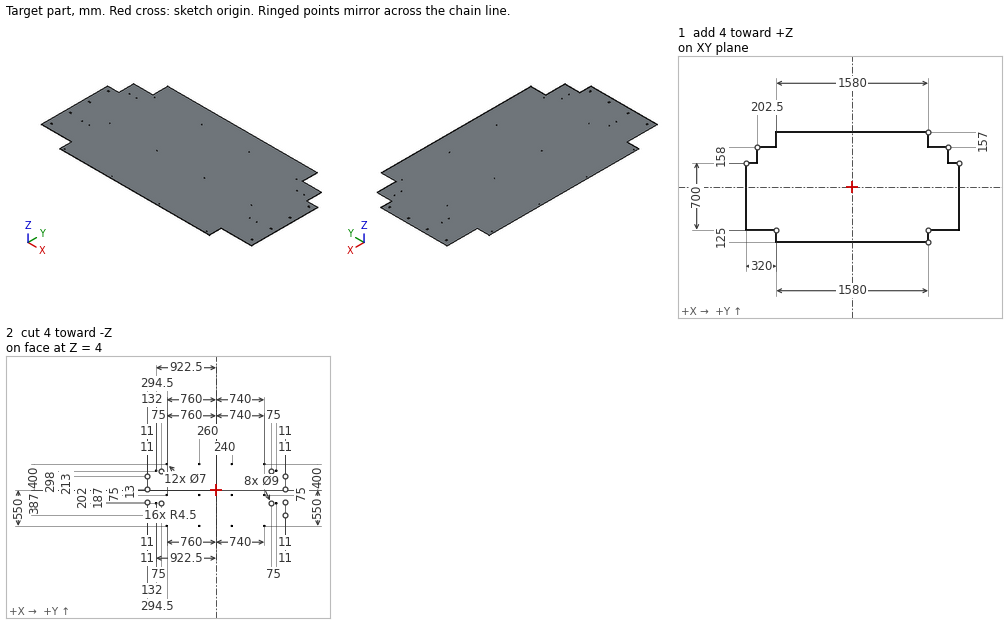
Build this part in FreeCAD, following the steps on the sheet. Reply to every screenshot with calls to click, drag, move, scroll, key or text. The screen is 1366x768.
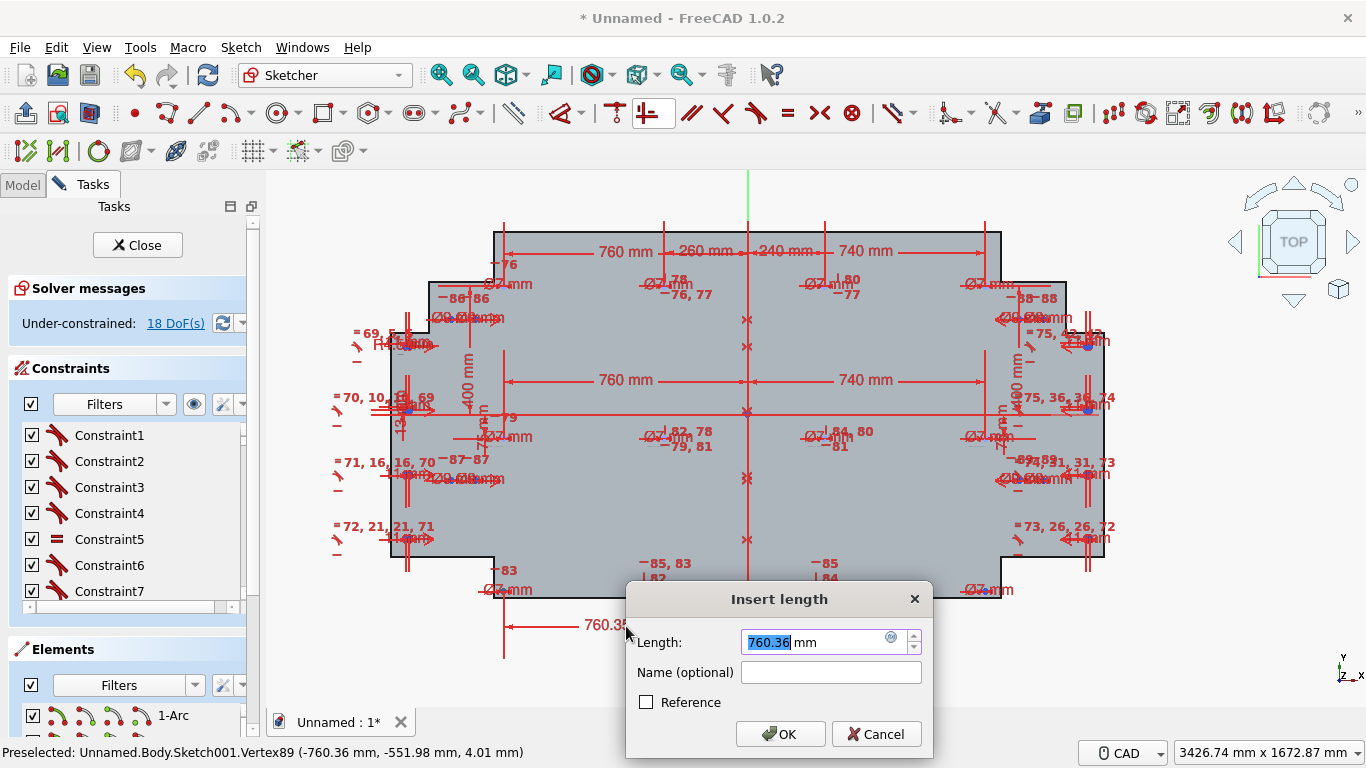
text(760)
key(Return)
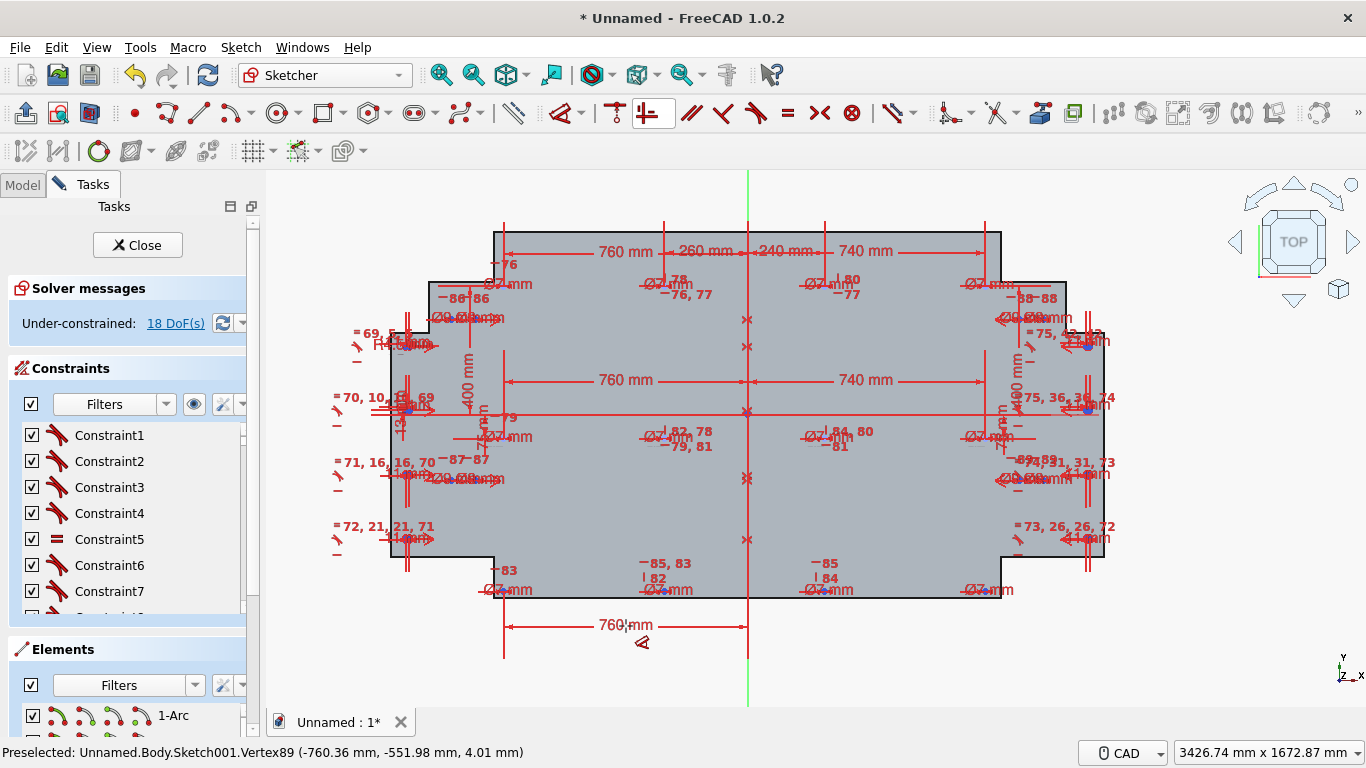
click(504, 592)
click(470, 503)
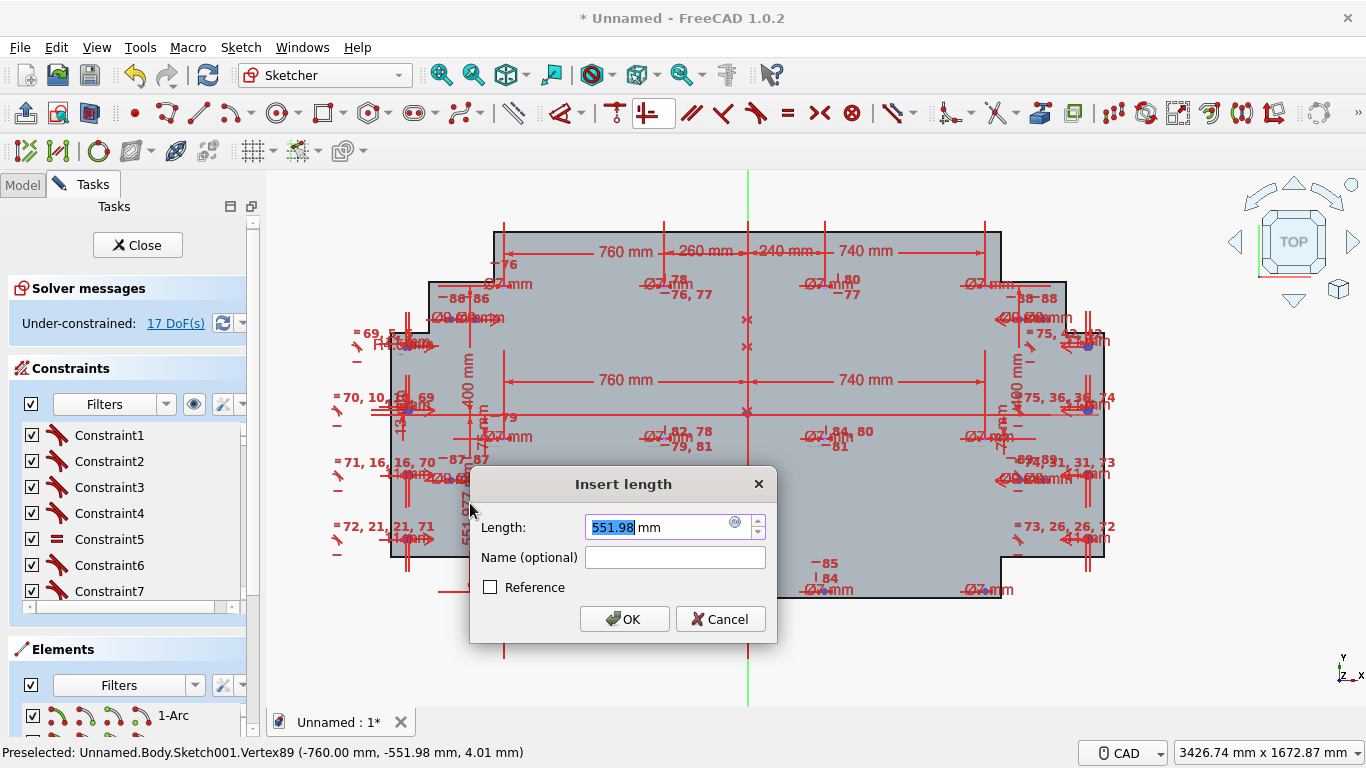
text(550)
key(Return)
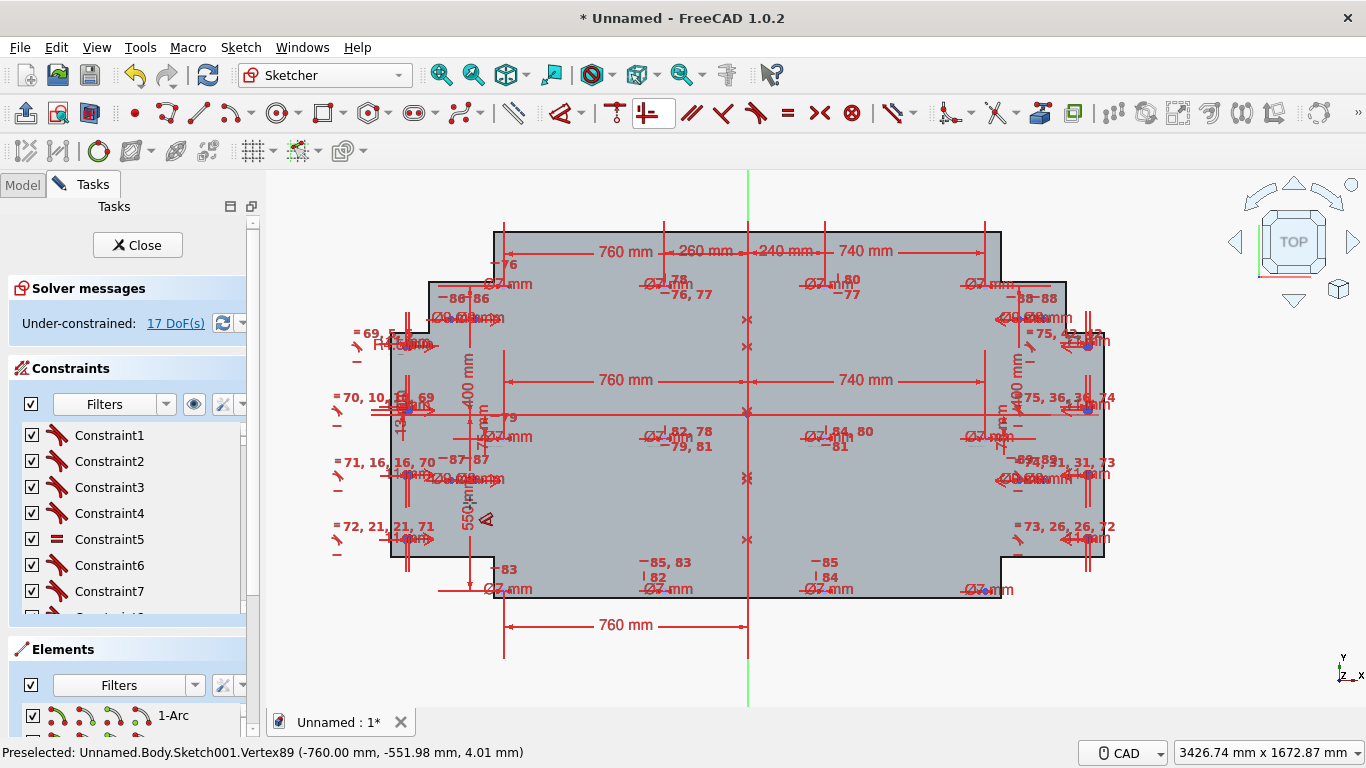
click(985, 592)
click(866, 626)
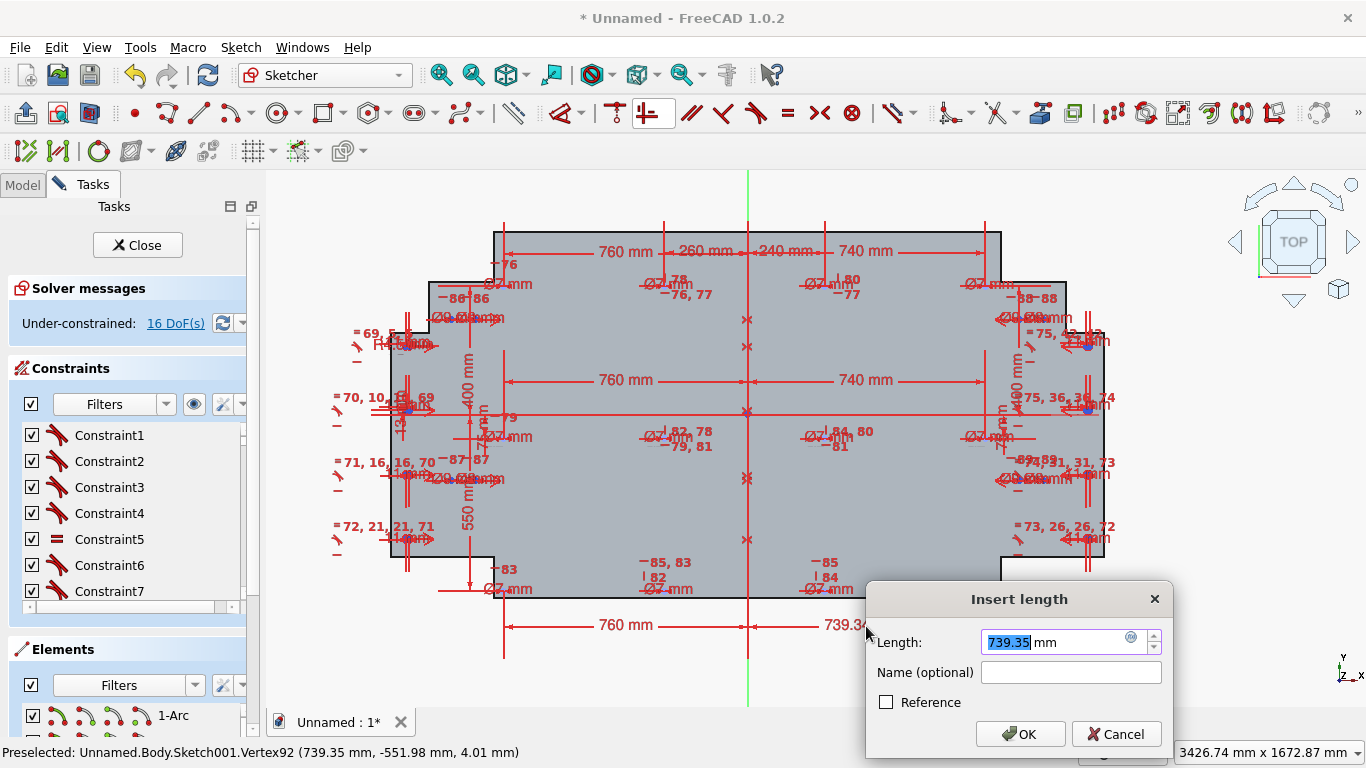
text(740)
key(Return)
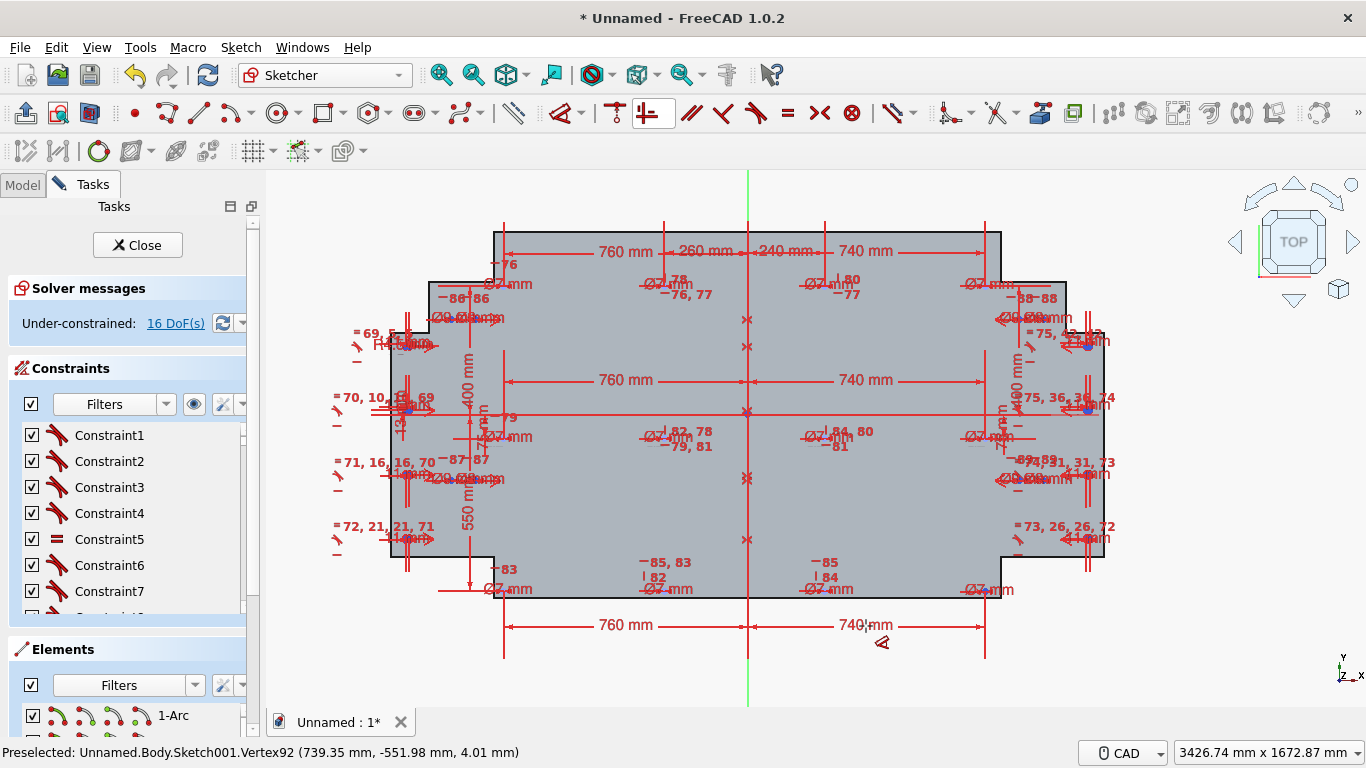
click(985, 592)
click(1019, 503)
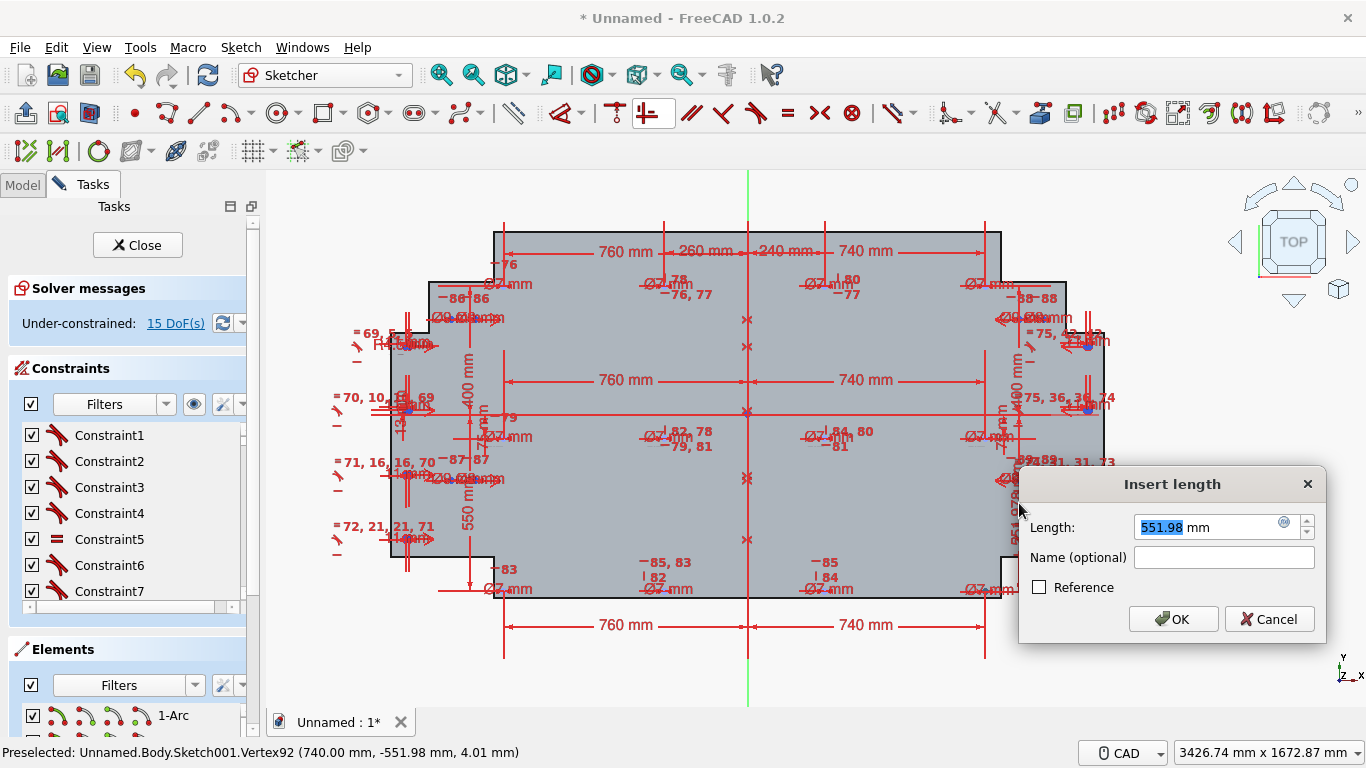
text(550)
key(Return)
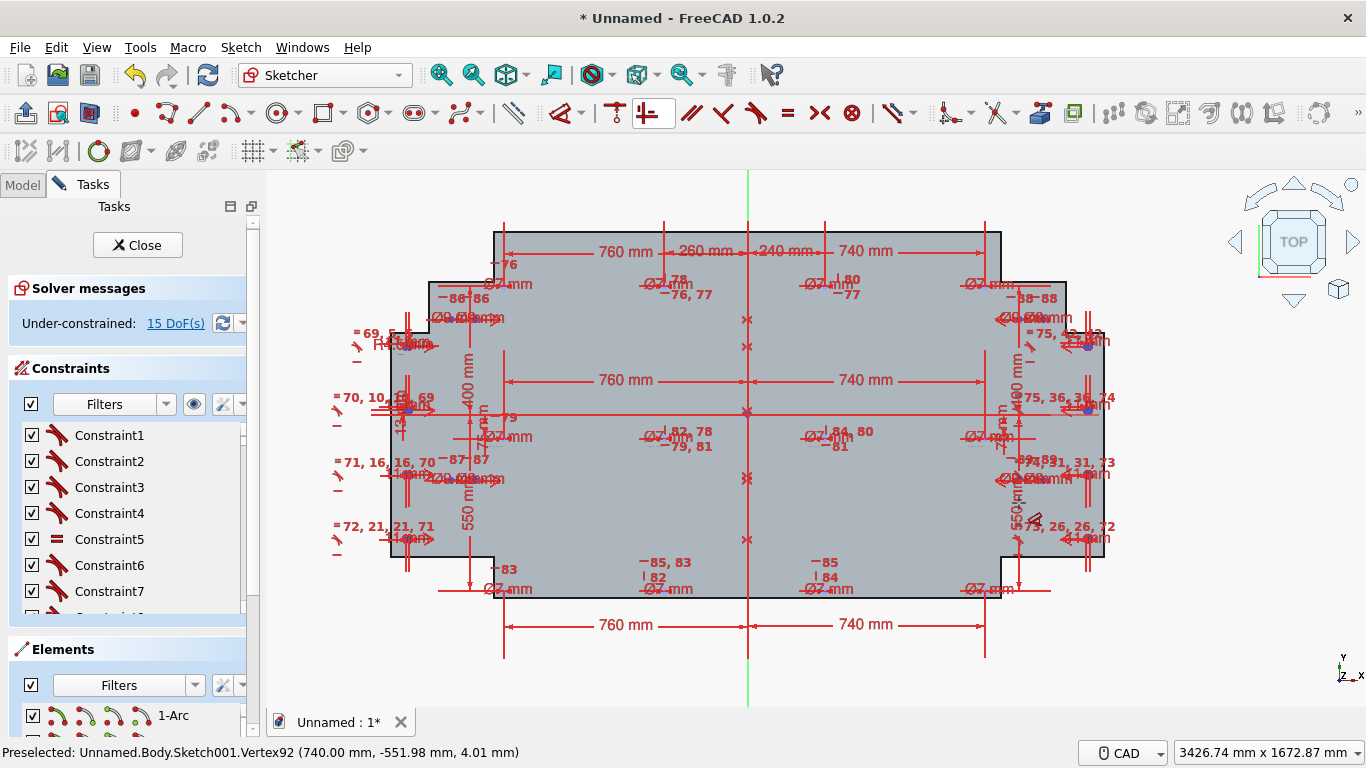
click(451, 320)
click(782, 367)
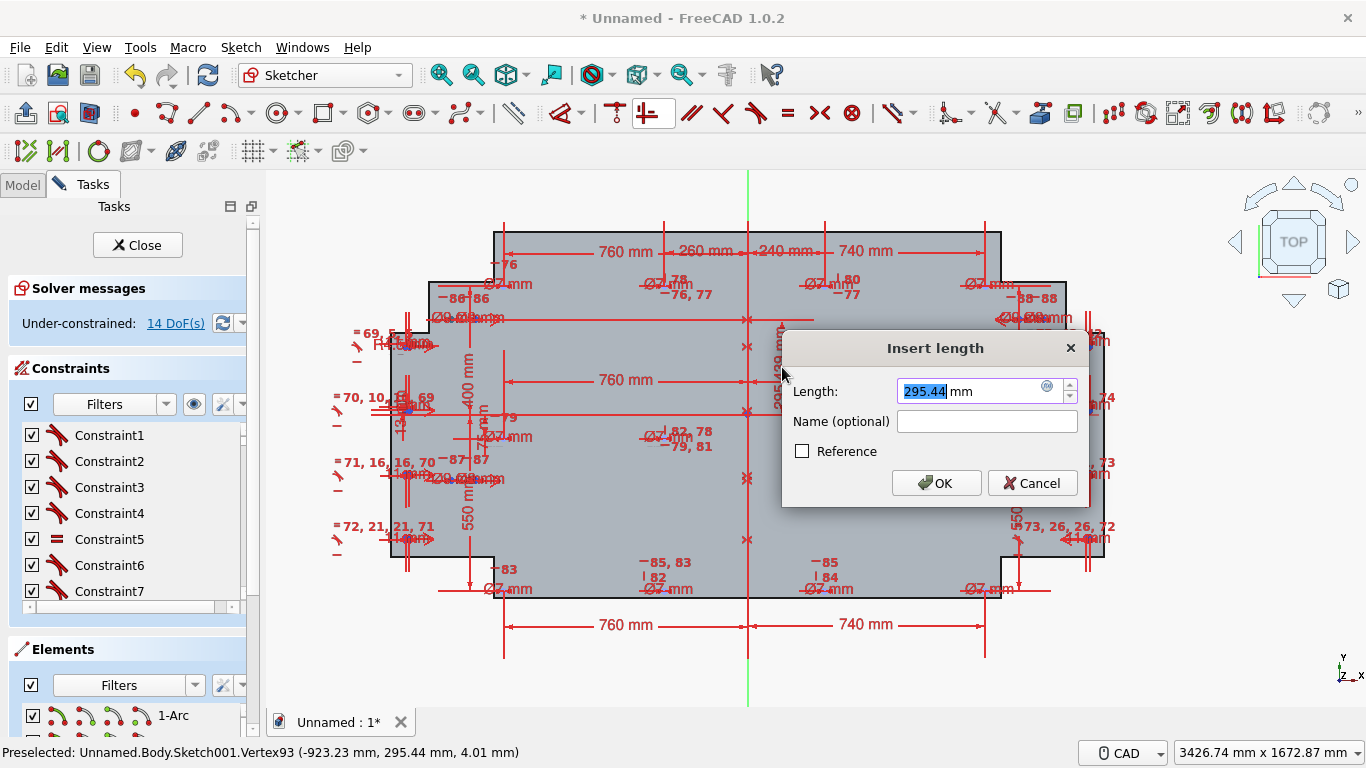
text(298)
key(Return)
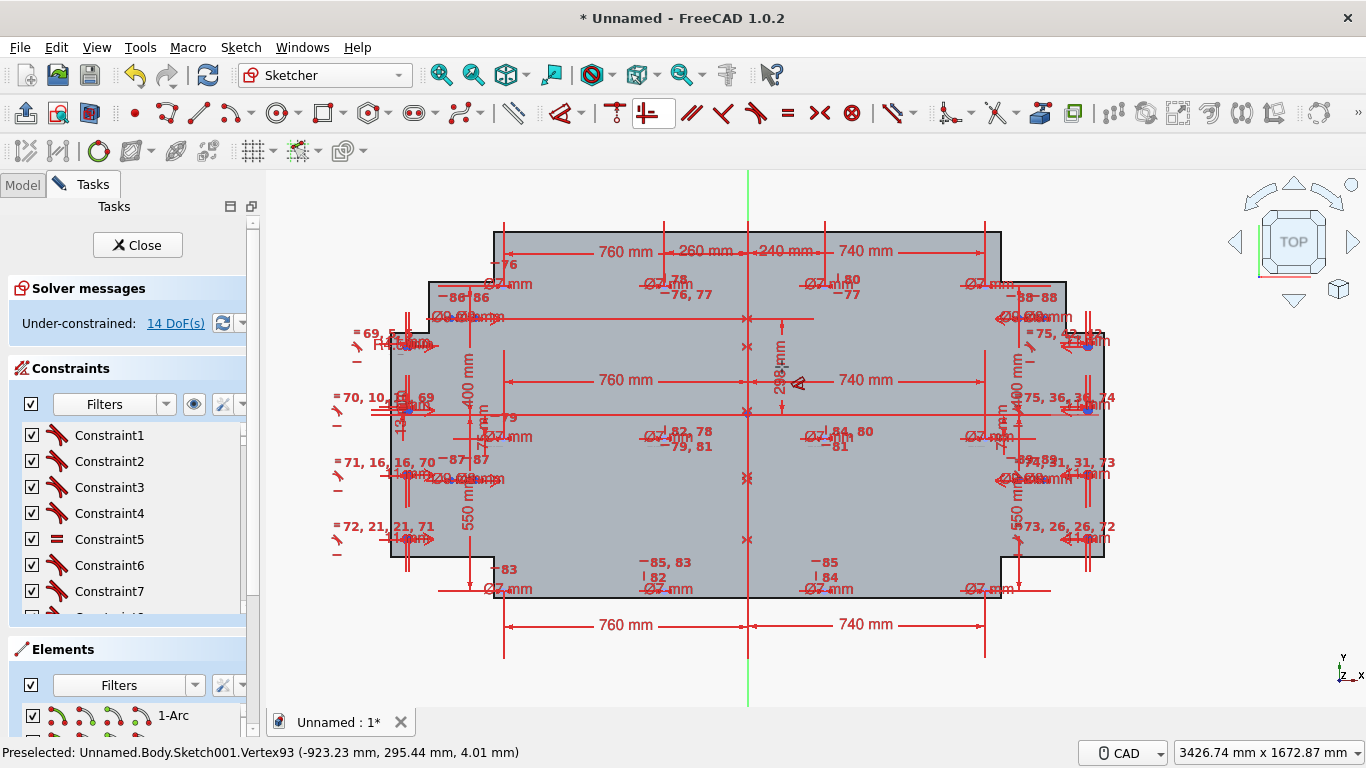
click(451, 481)
click(417, 448)